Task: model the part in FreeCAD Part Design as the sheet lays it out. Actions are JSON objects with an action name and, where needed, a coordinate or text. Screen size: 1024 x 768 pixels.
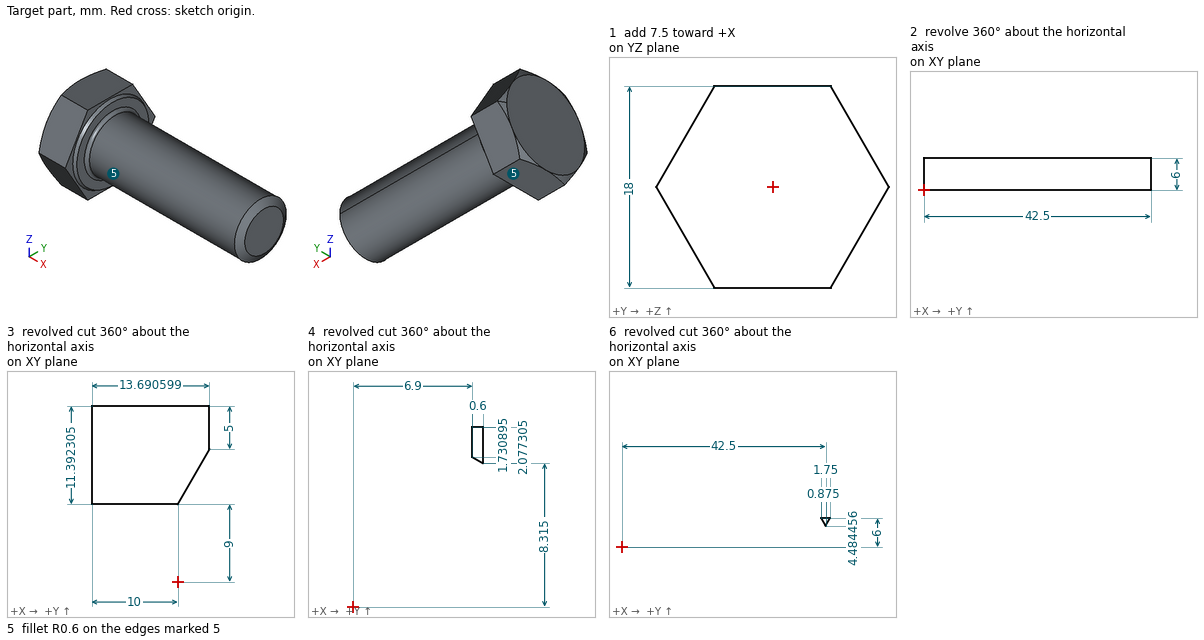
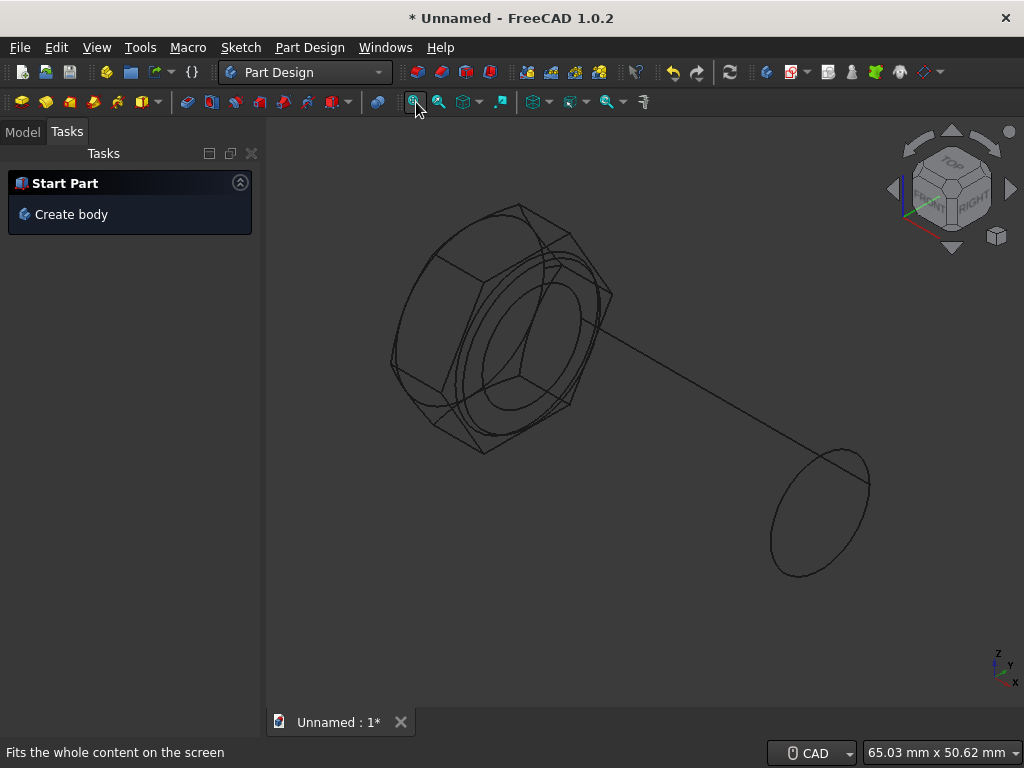
{"action": "left_click", "coordinate": [482, 374]}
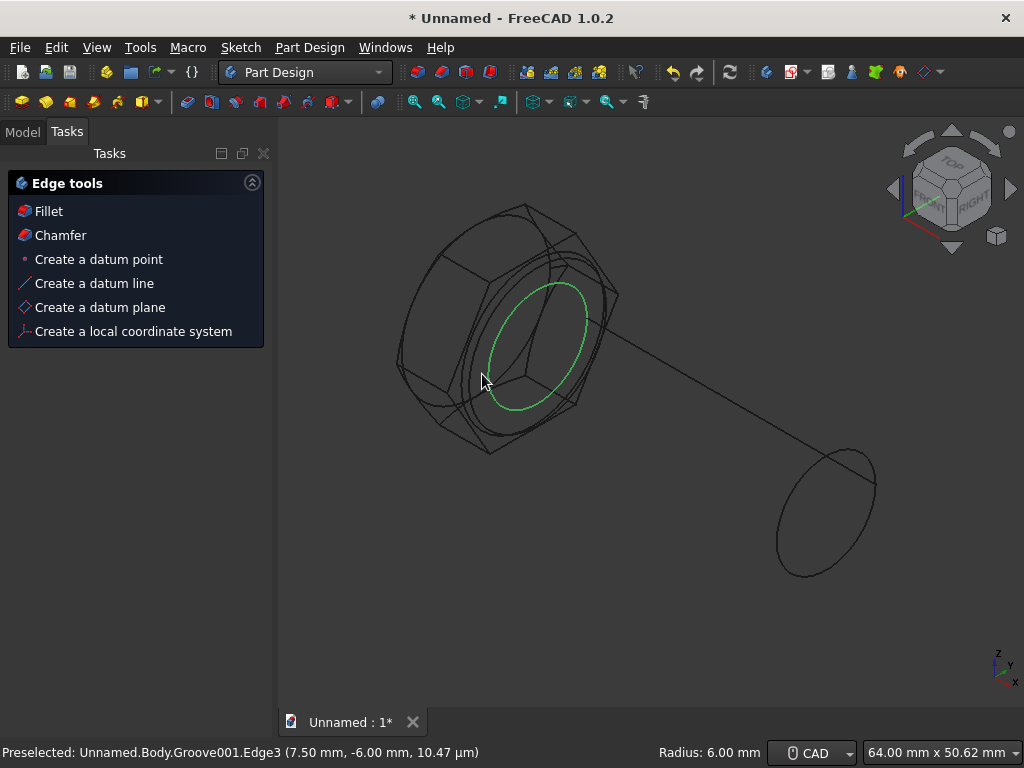
{"action": "key", "text": "v 1"}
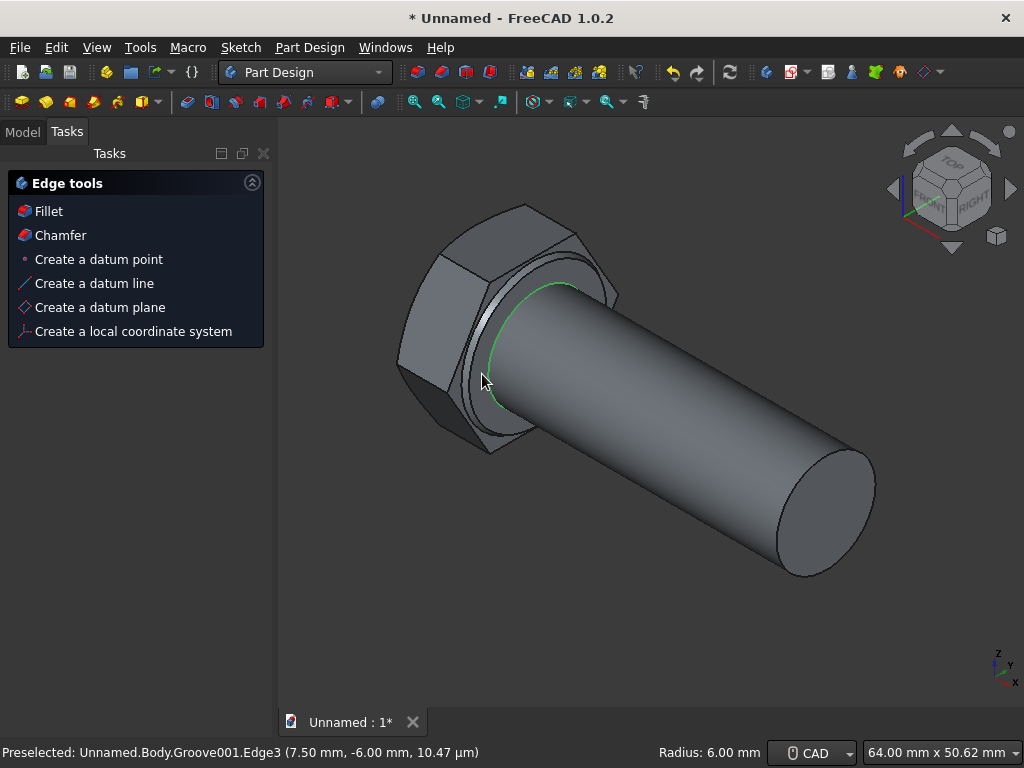
{"action": "left_click", "coordinate": [418, 72]}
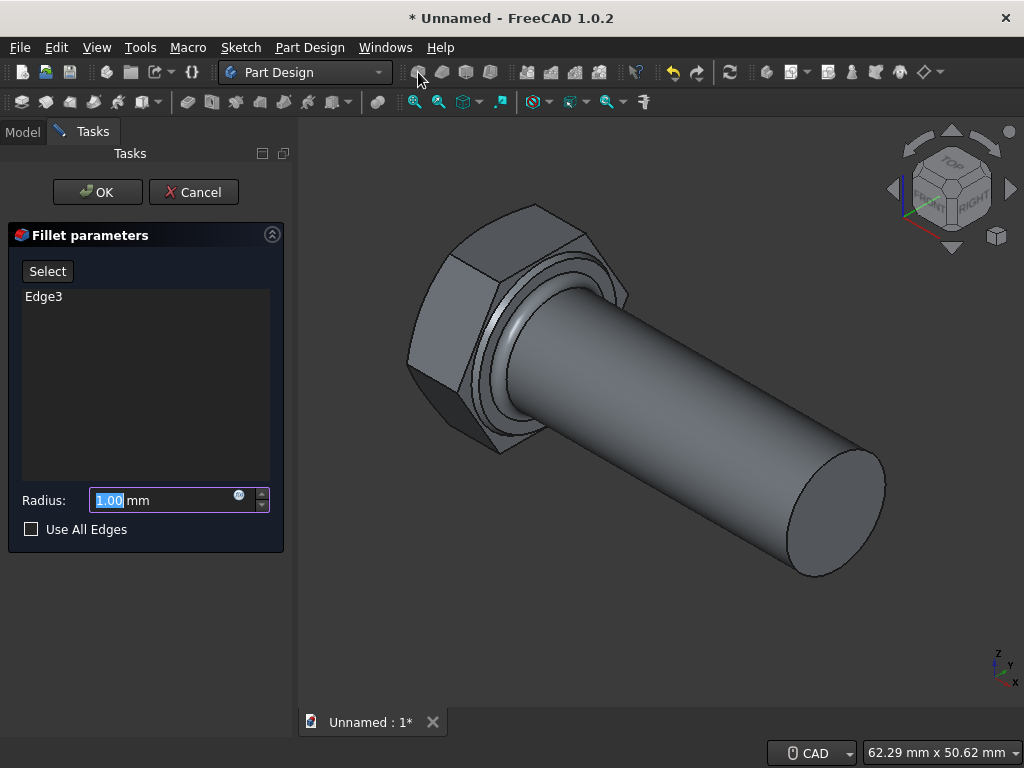
{"action": "type", "text": "0.6"}
{"action": "key", "text": "Tab"}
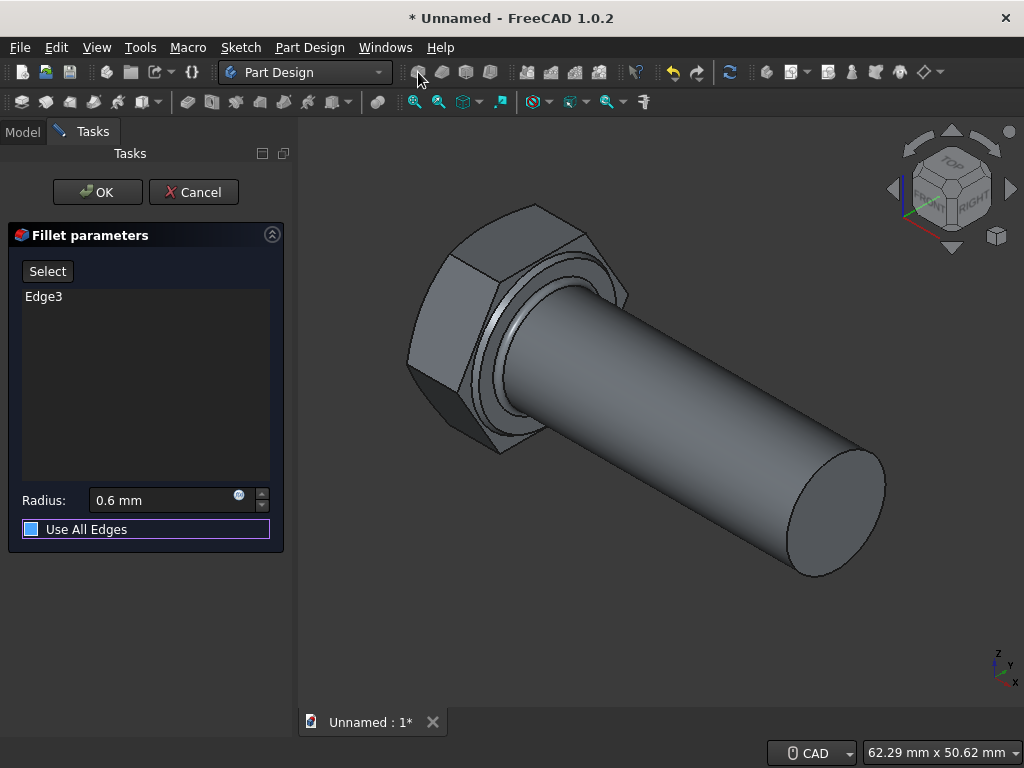
{"action": "left_click", "coordinate": [98, 192]}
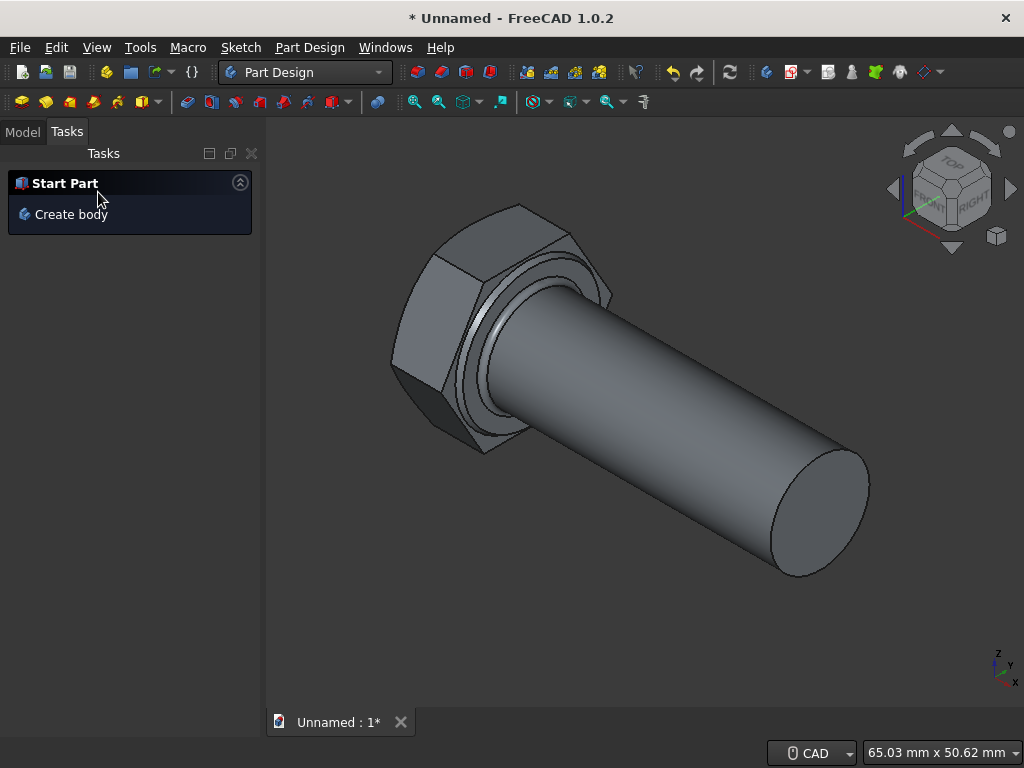
{"action": "left_click", "coordinate": [792, 72]}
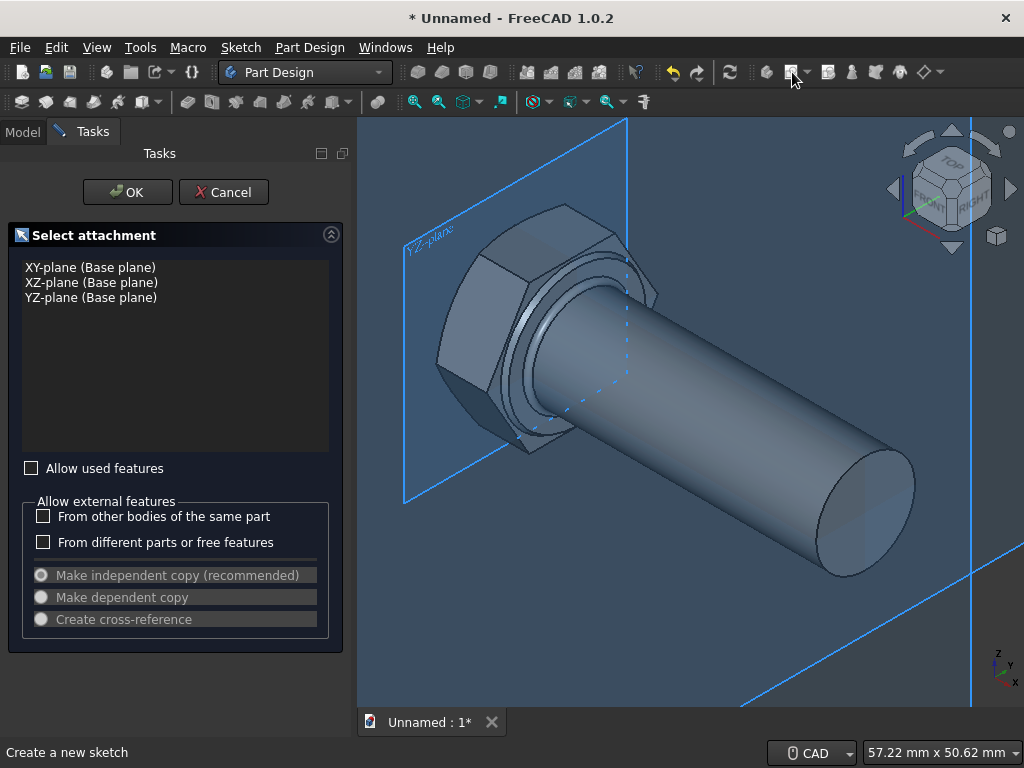
{"action": "left_click", "coordinate": [82, 268]}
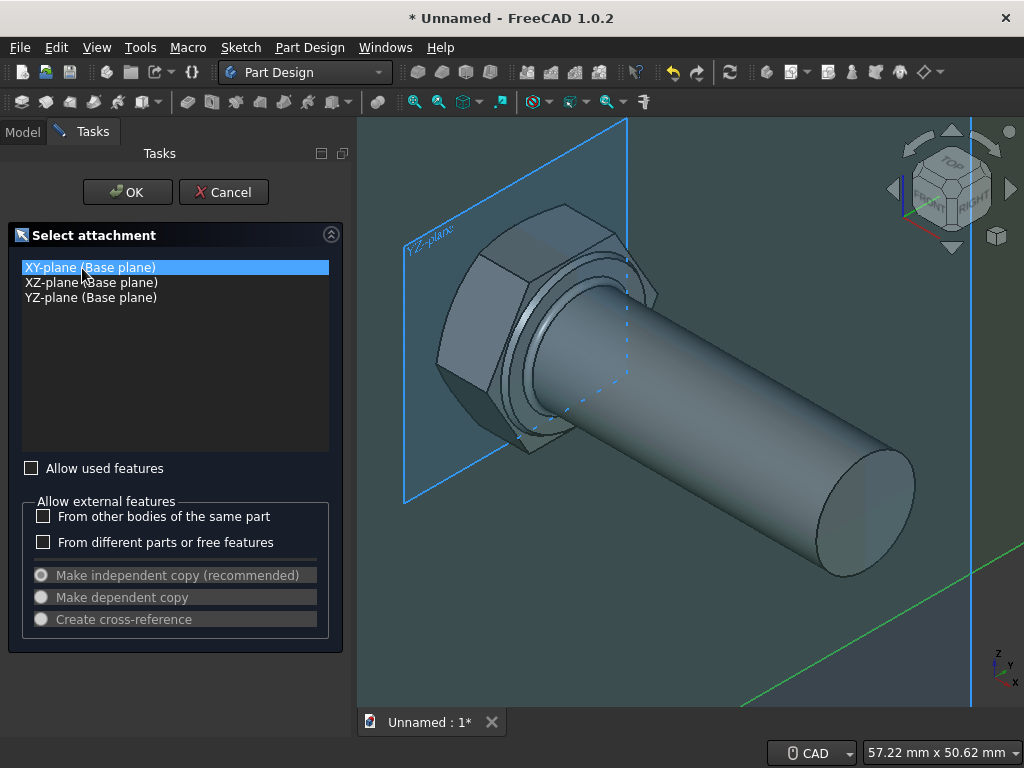
{"action": "left_click", "coordinate": [128, 192]}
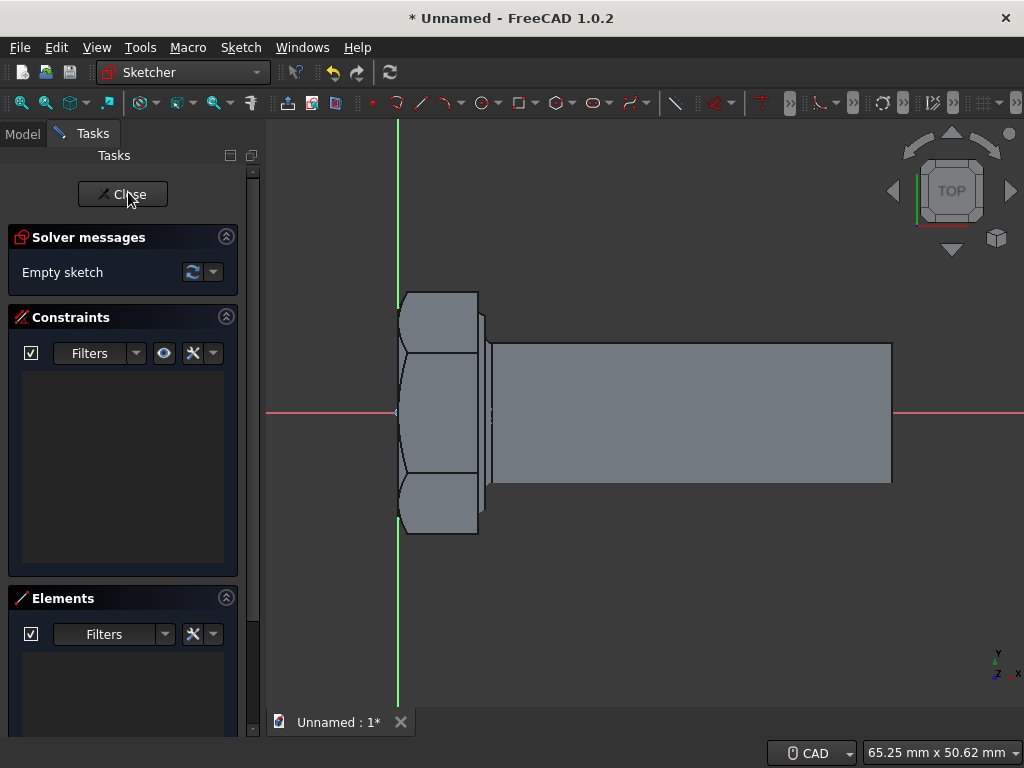
{"action": "left_click", "coordinate": [336, 104]}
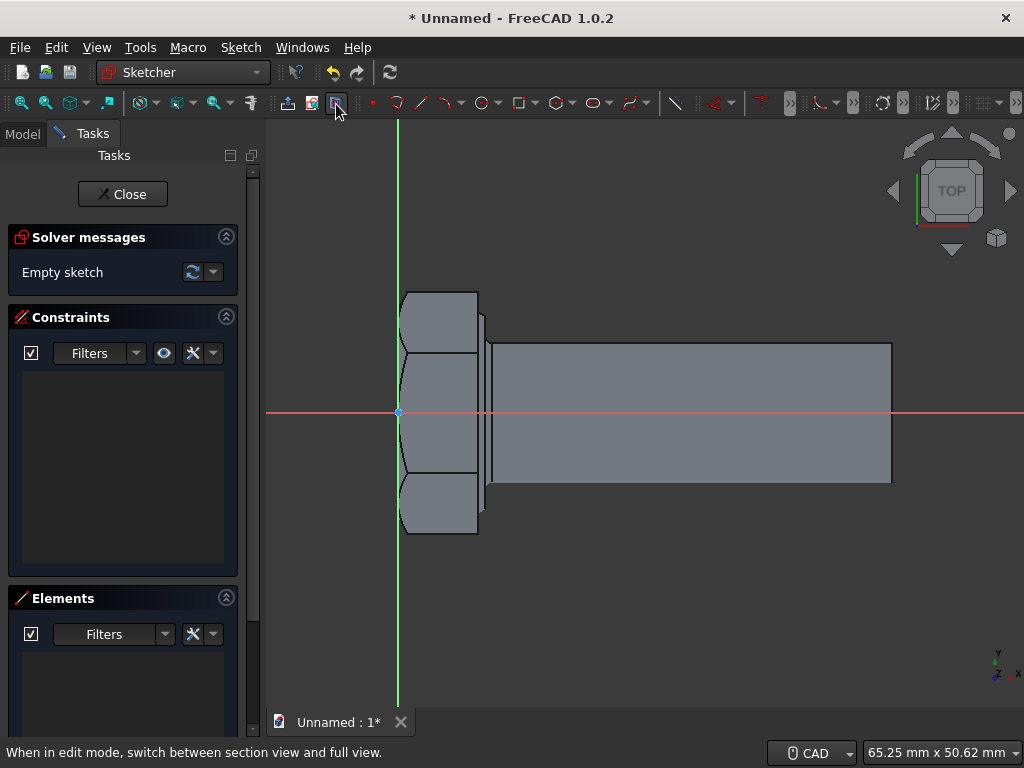
{"action": "scroll", "coordinate": [576, 413], "scroll_direction": "down", "scroll_amount": 5}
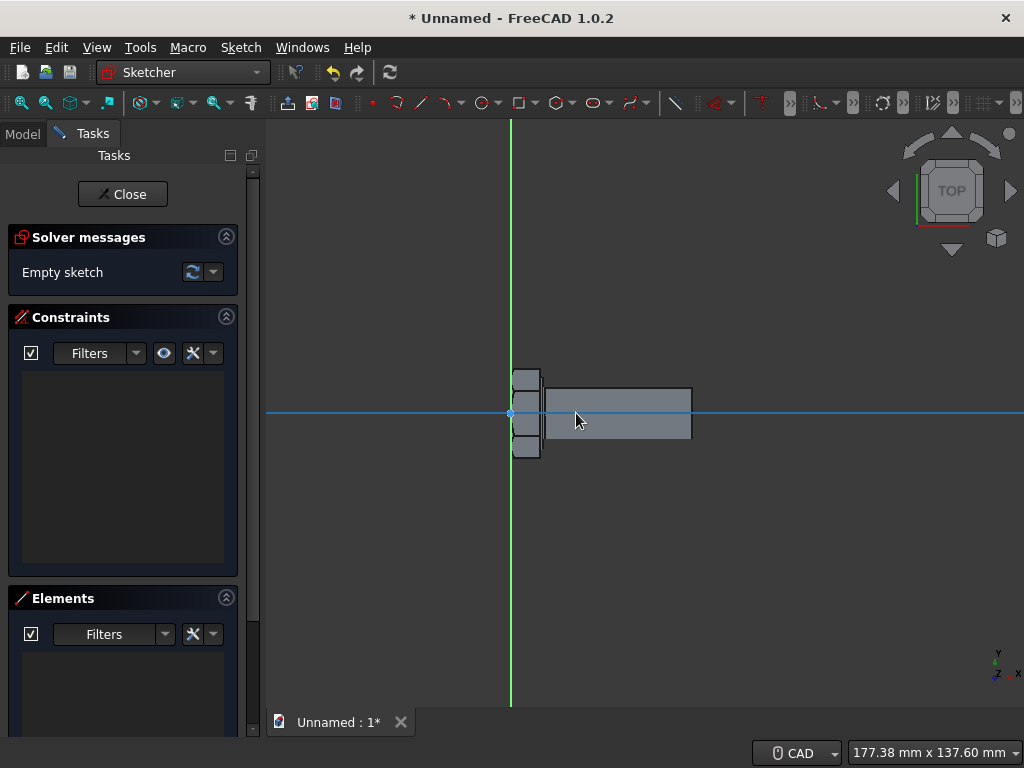
{"action": "scroll", "coordinate": [699, 390], "scroll_direction": "up", "scroll_amount": 15}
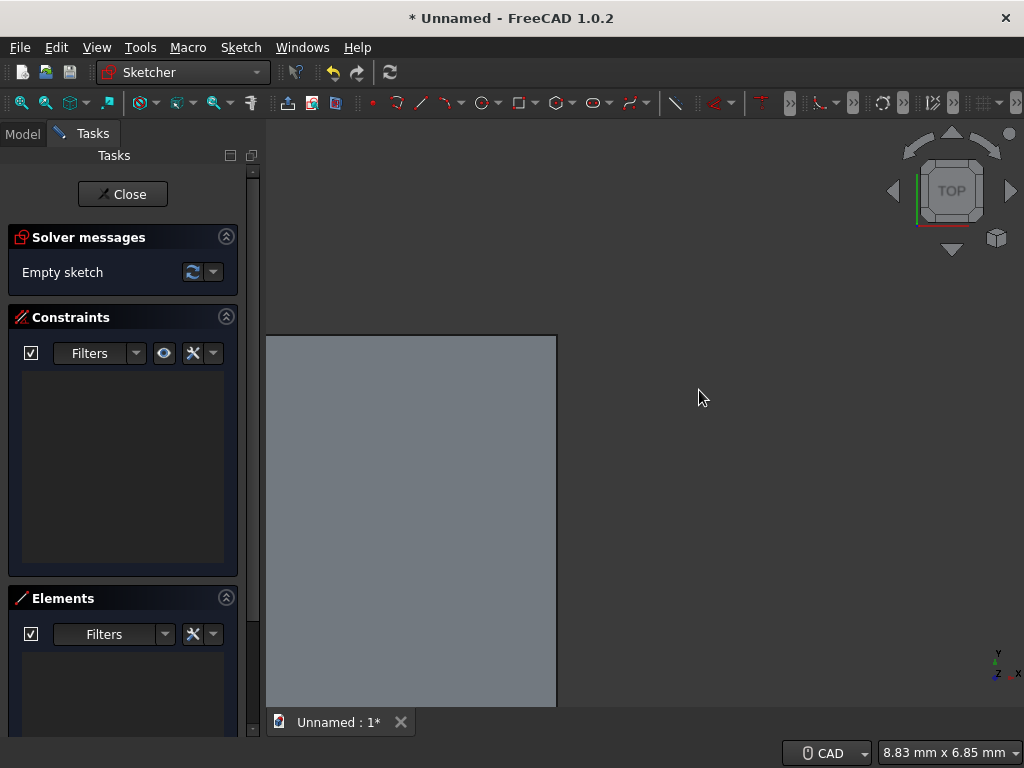
{"action": "scroll", "coordinate": [545, 392], "scroll_direction": "up", "scroll_amount": 5}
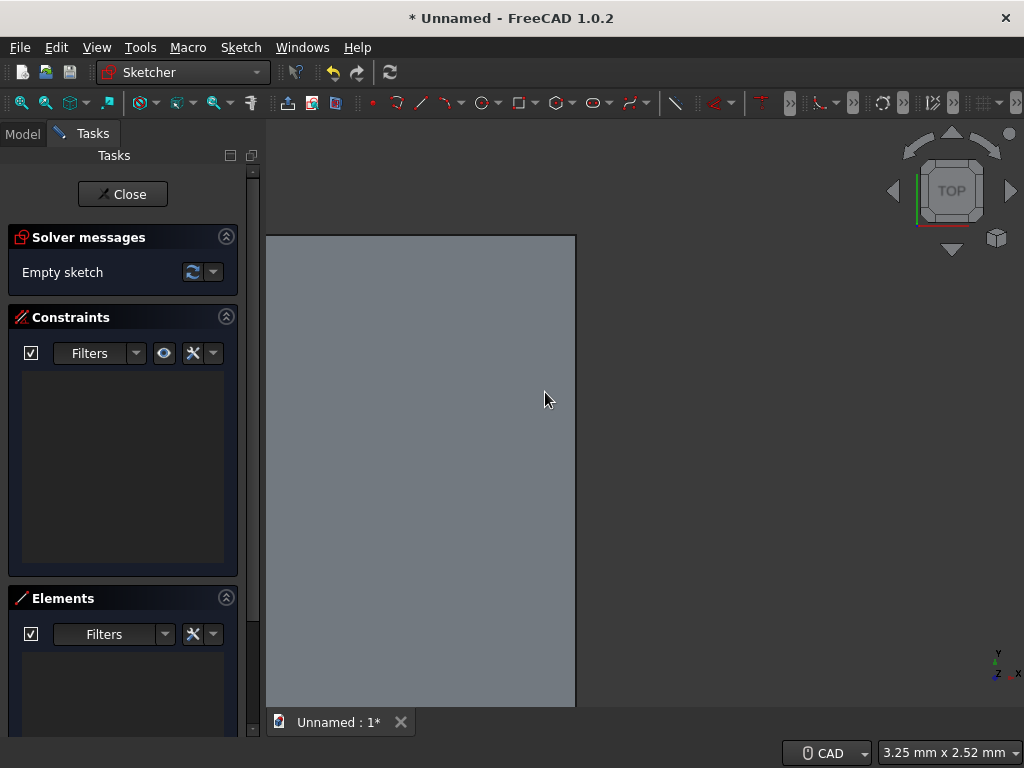
{"action": "left_click", "coordinate": [398, 104]}